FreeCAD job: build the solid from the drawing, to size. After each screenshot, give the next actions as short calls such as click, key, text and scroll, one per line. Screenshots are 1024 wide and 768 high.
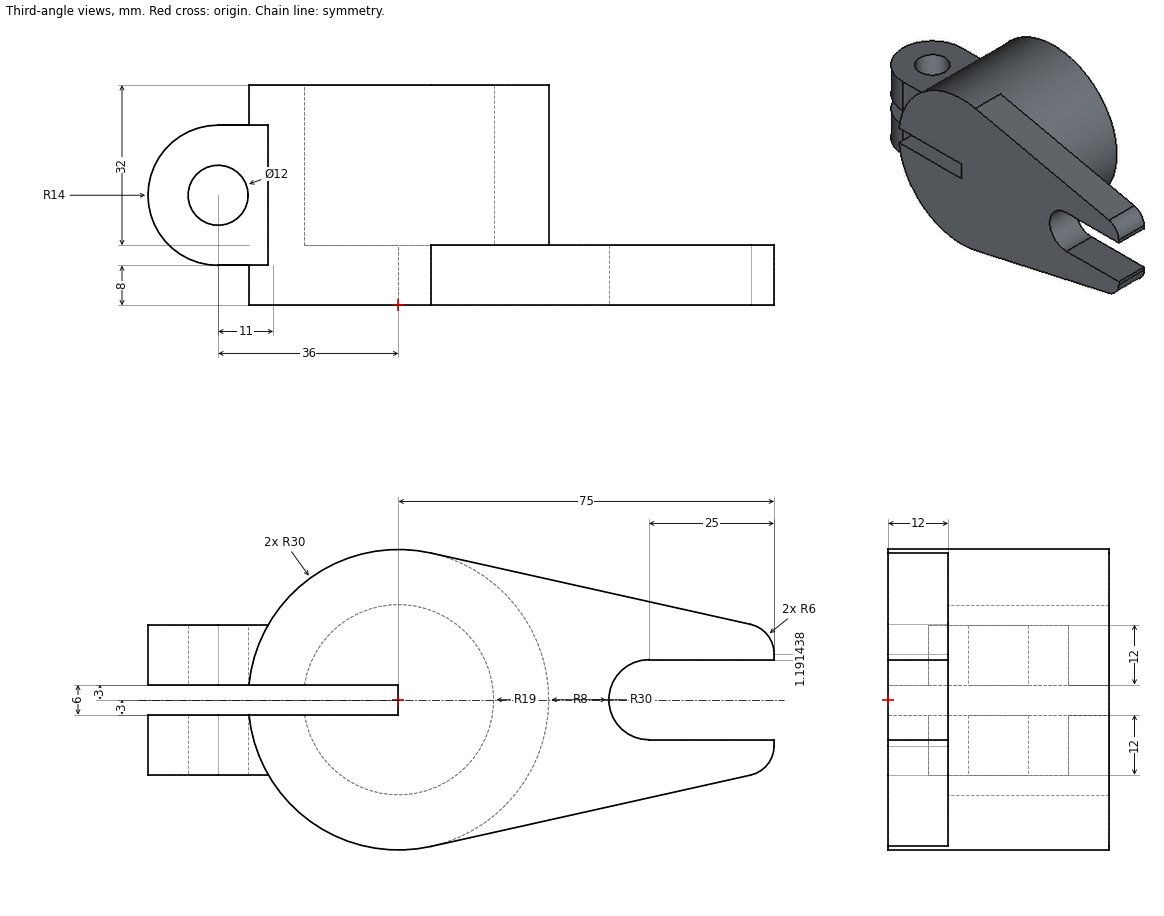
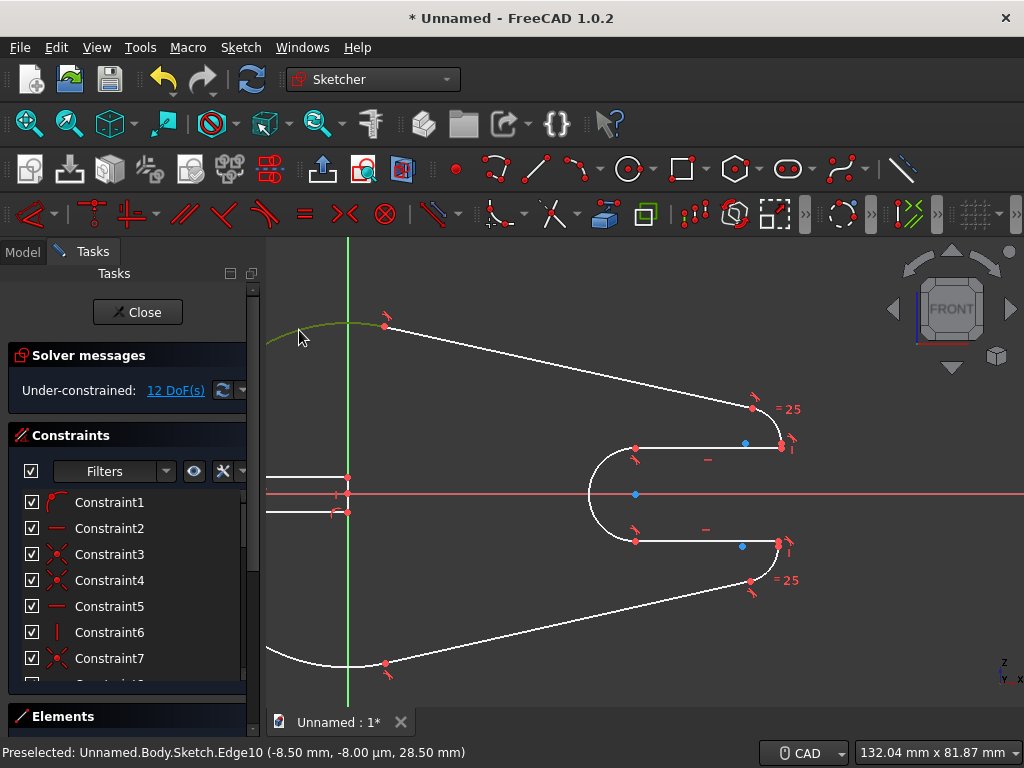
click(299, 660)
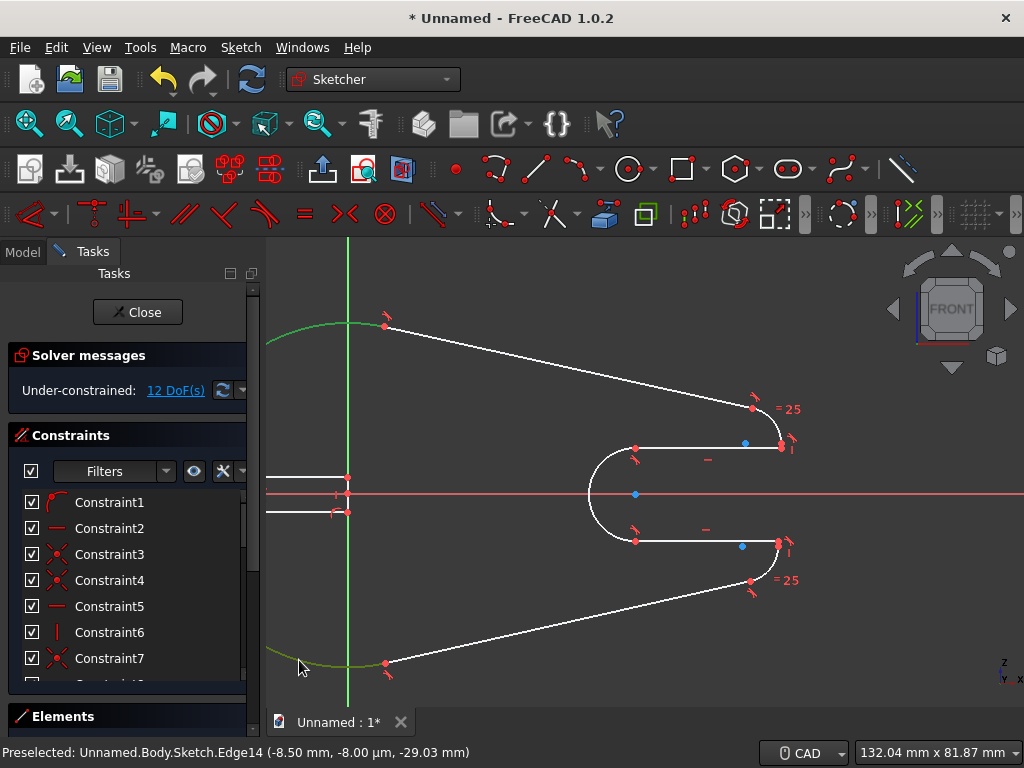
key(e)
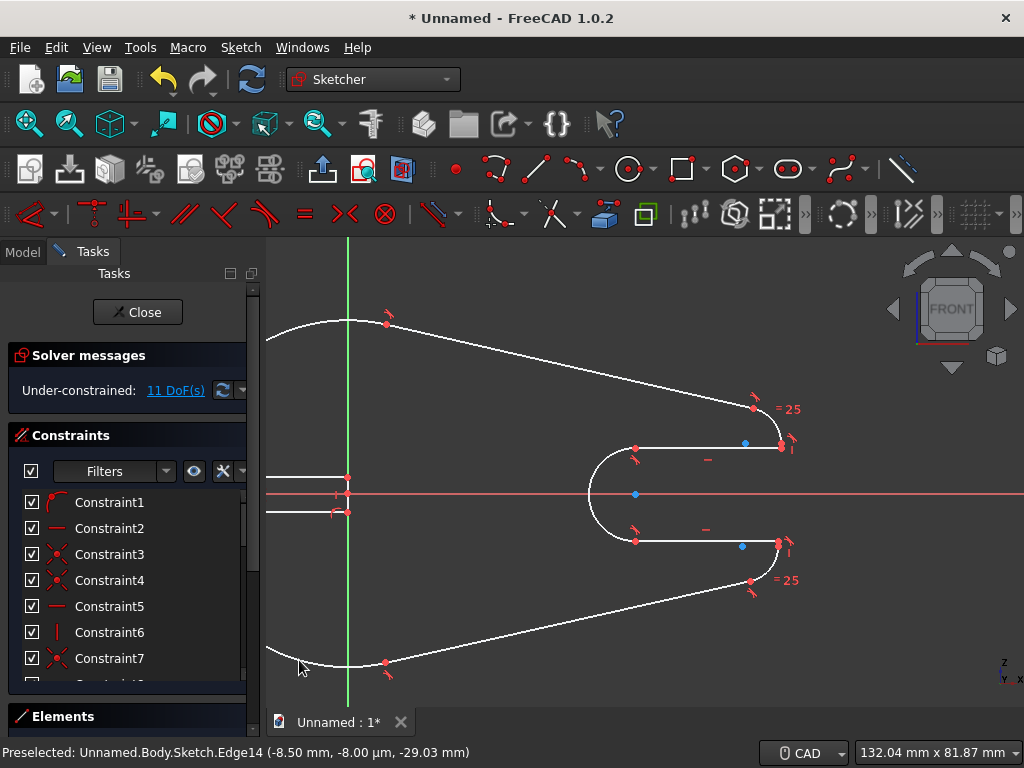
click(636, 495)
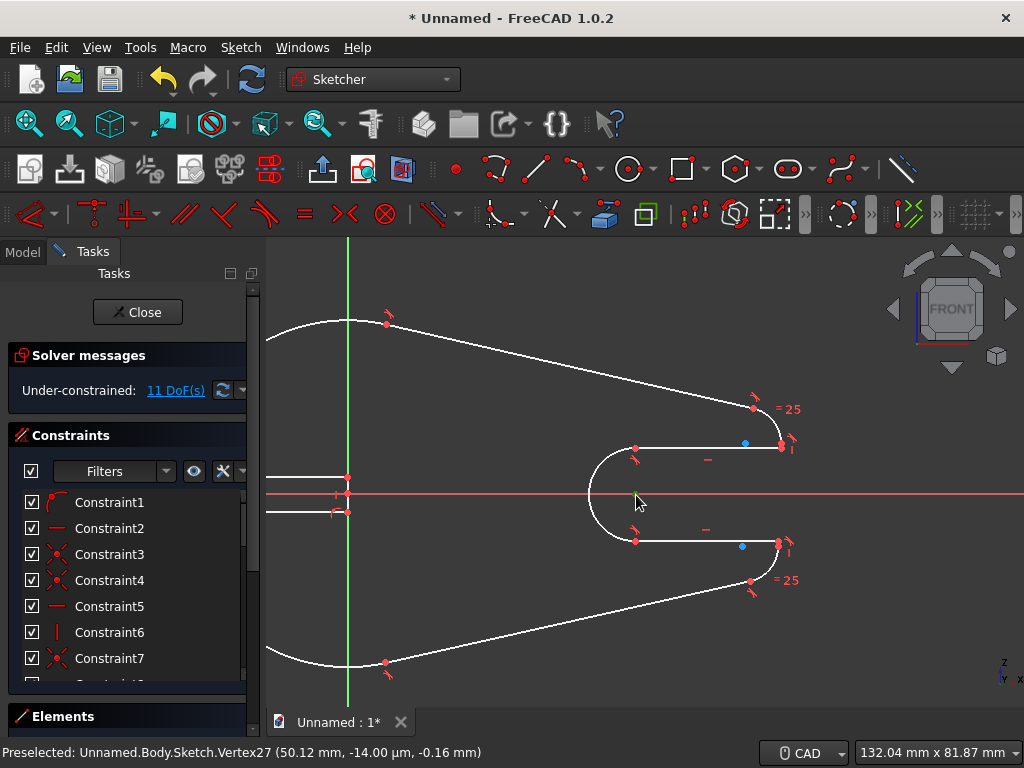
click(415, 494)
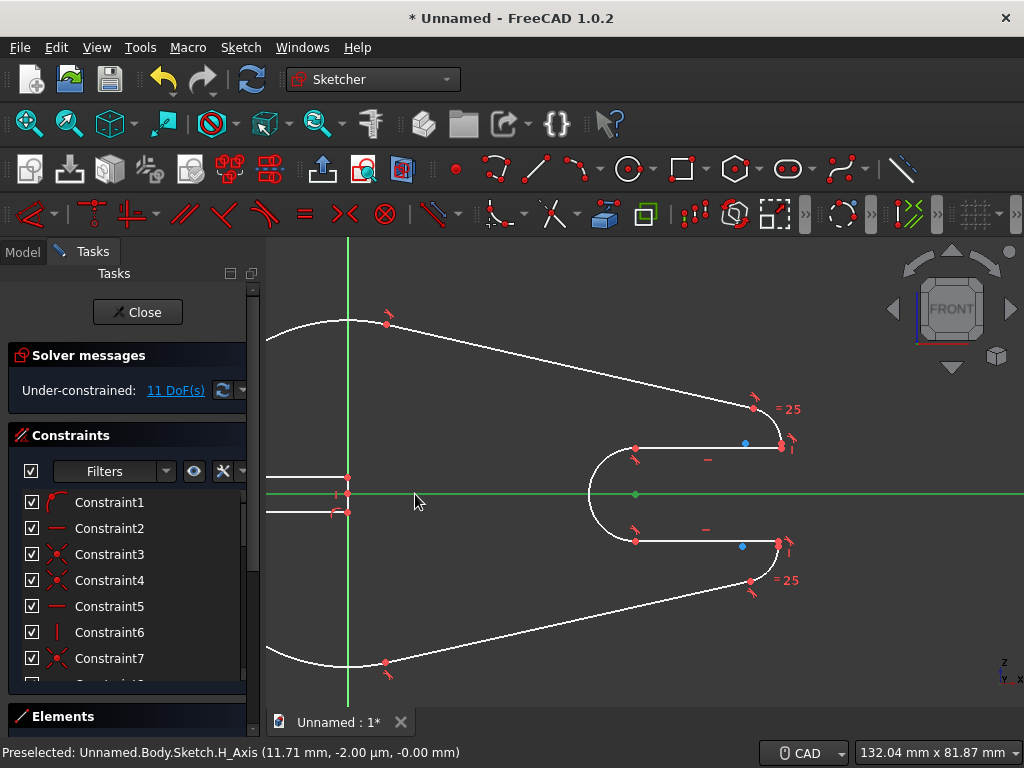
key(c)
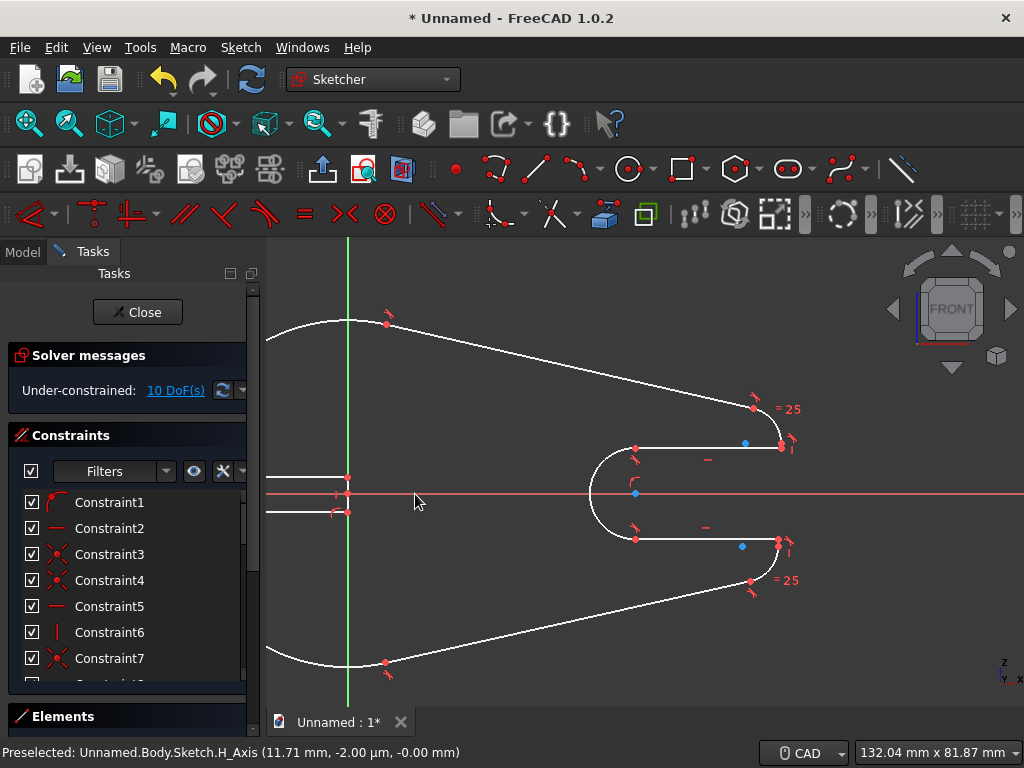
click(745, 444)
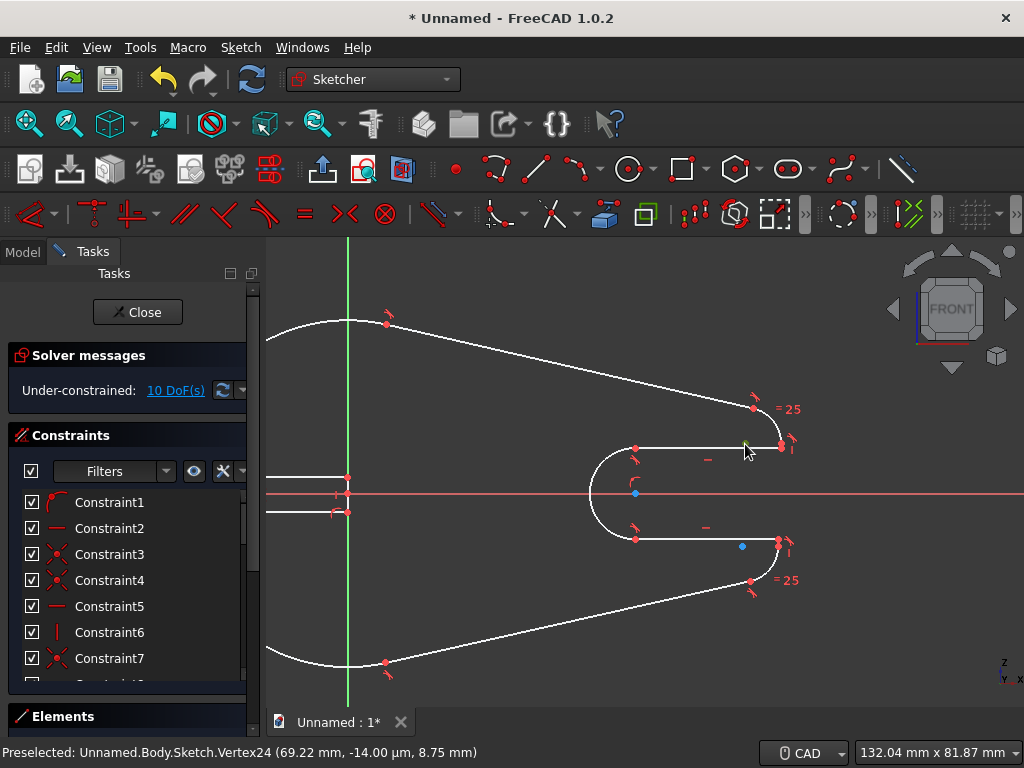
click(742, 546)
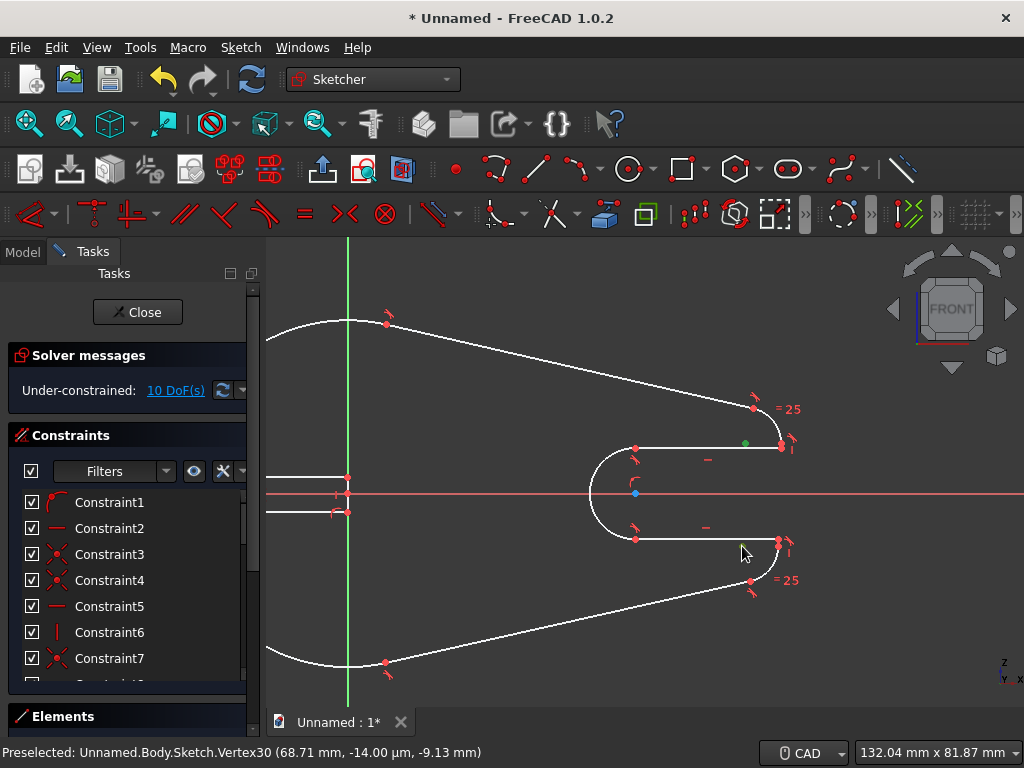
click(415, 494)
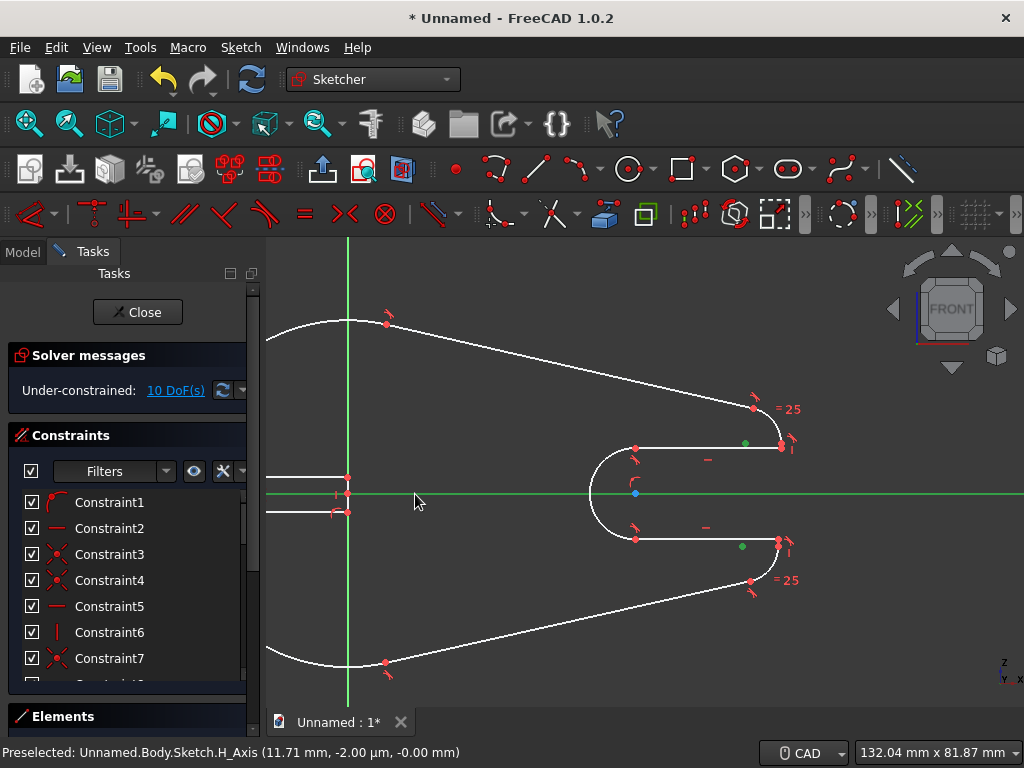
click(346, 214)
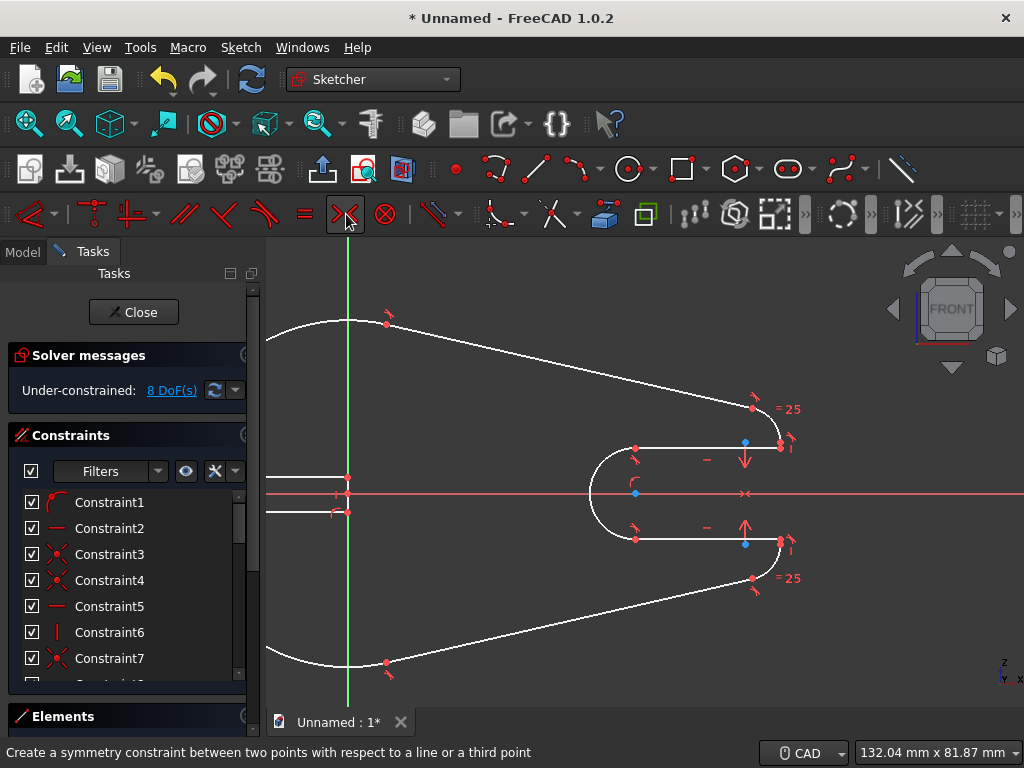
click(299, 327)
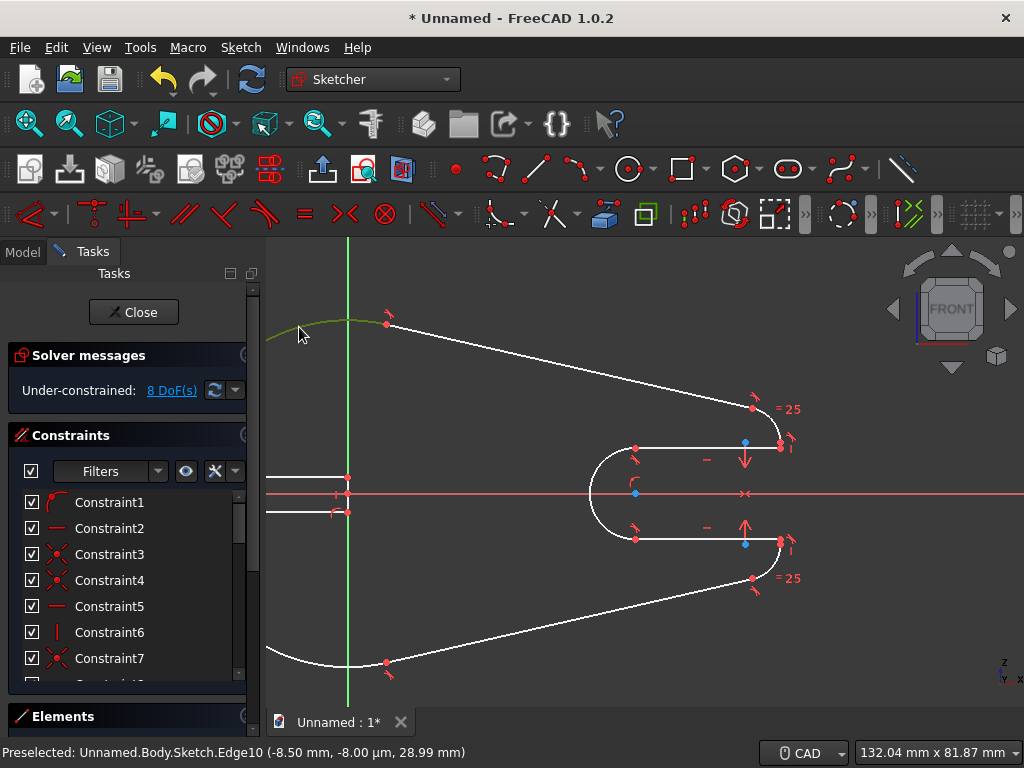
click(56, 214)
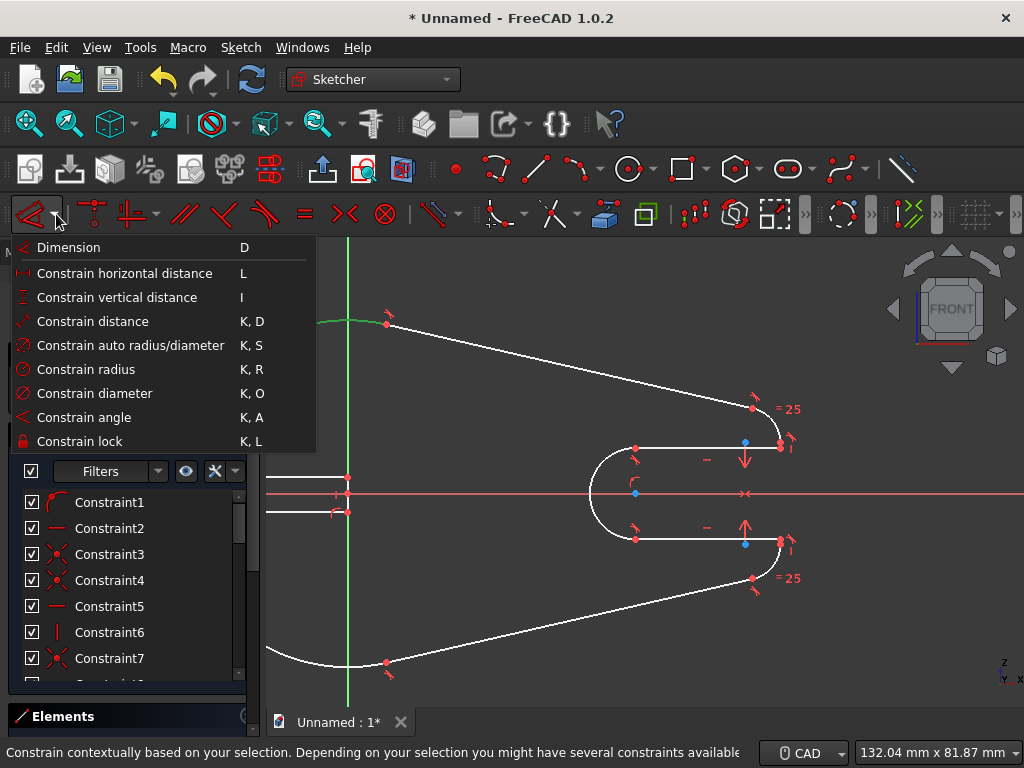
click(164, 369)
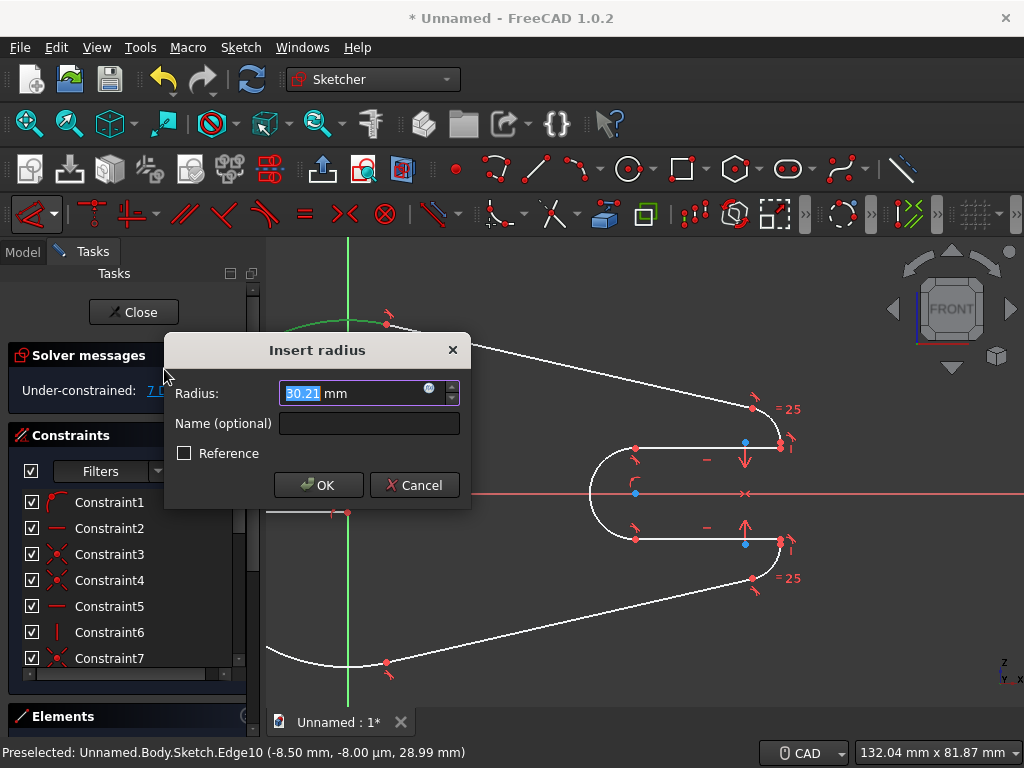
text(30)
key(Return)